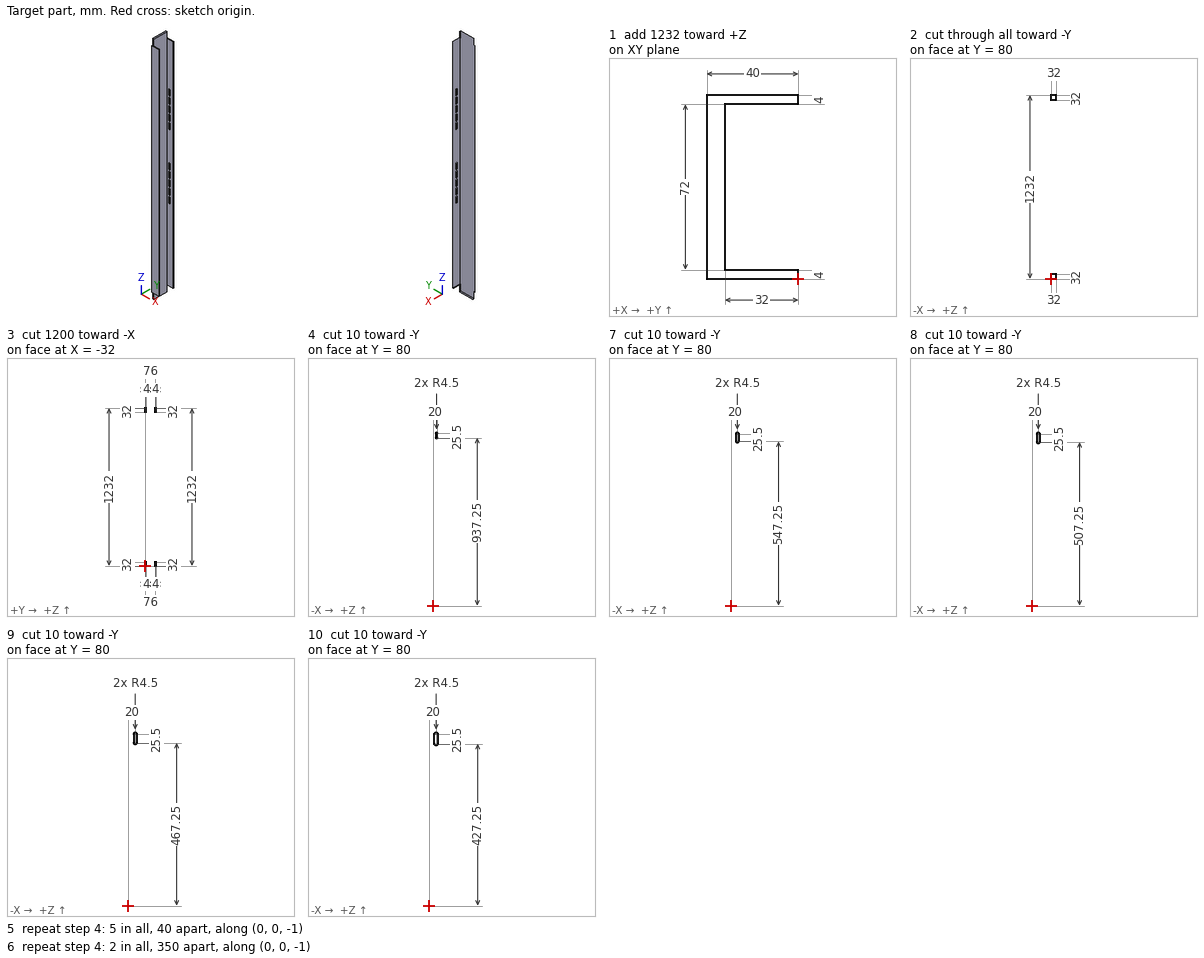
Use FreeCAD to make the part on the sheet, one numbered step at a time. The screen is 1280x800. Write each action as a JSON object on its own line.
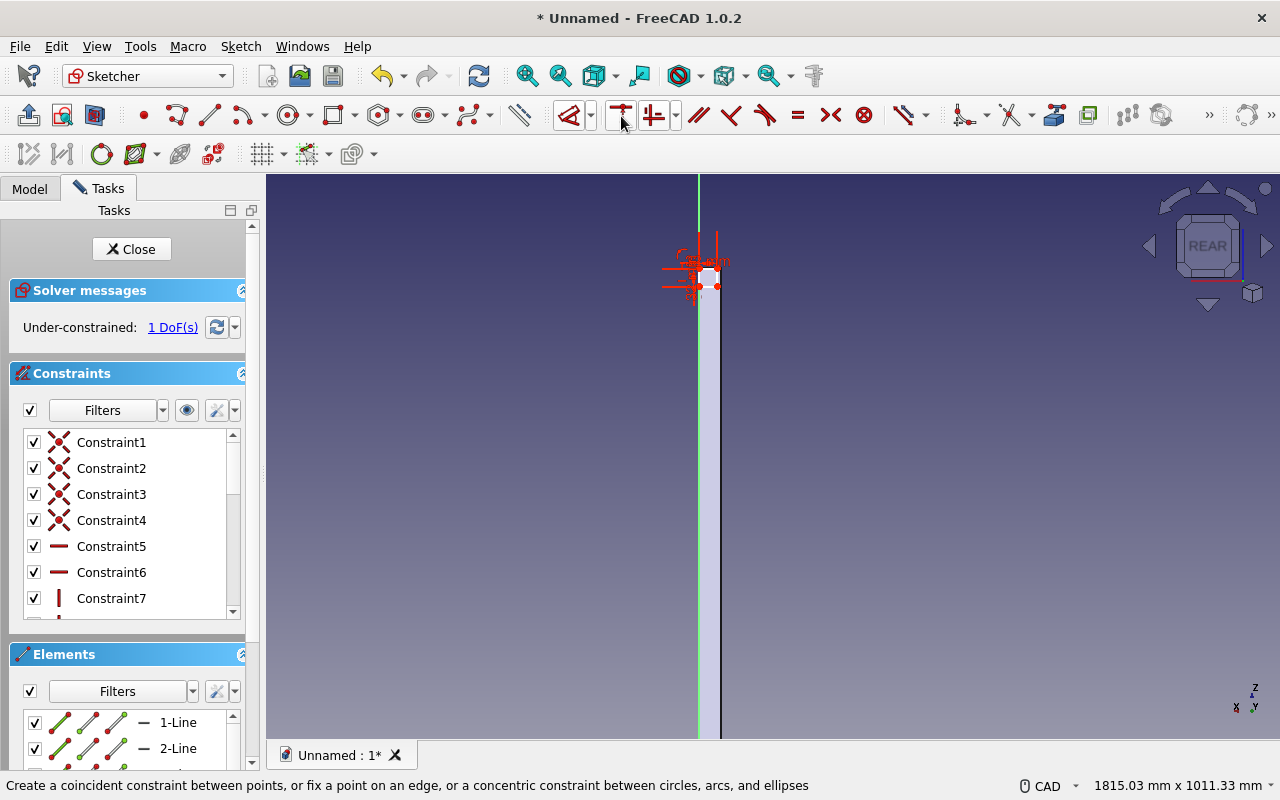
{"action": "left_click", "coordinate": [699, 269]}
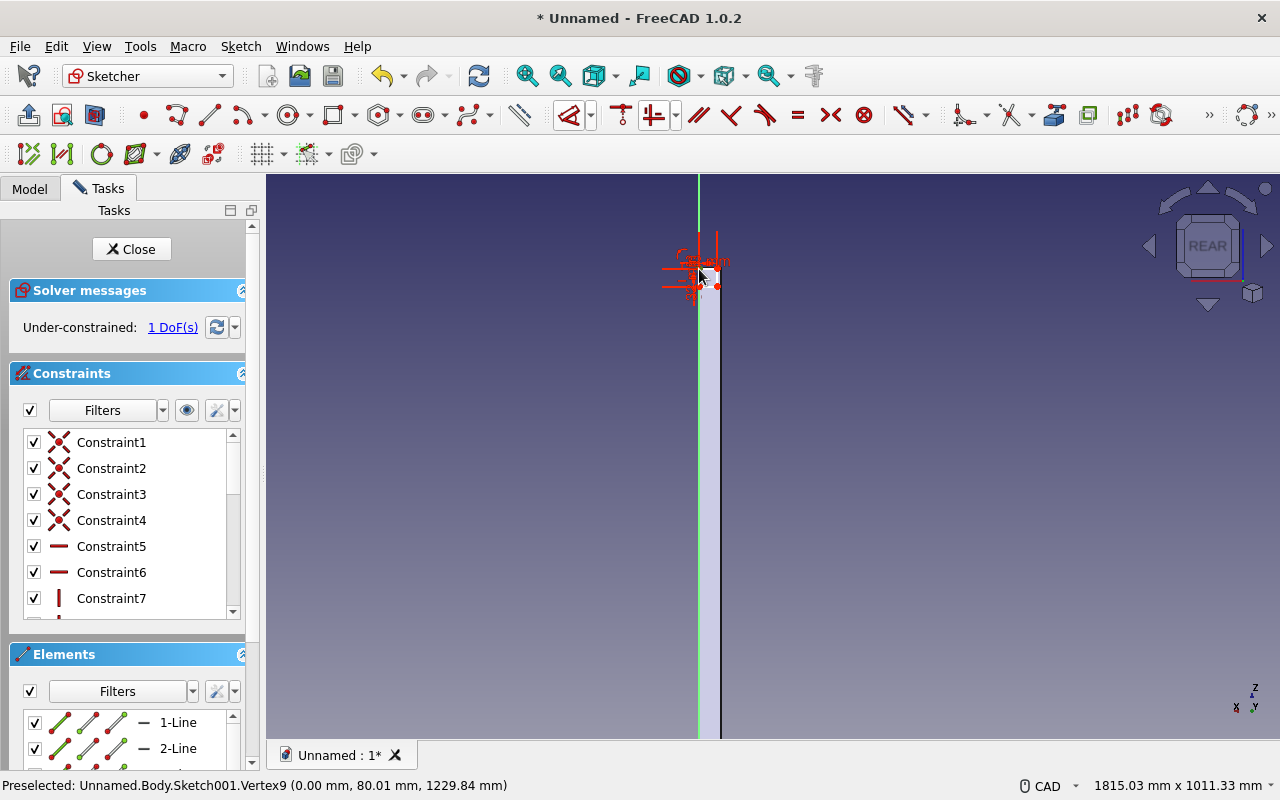
{"action": "left_click", "coordinate": [590, 116]}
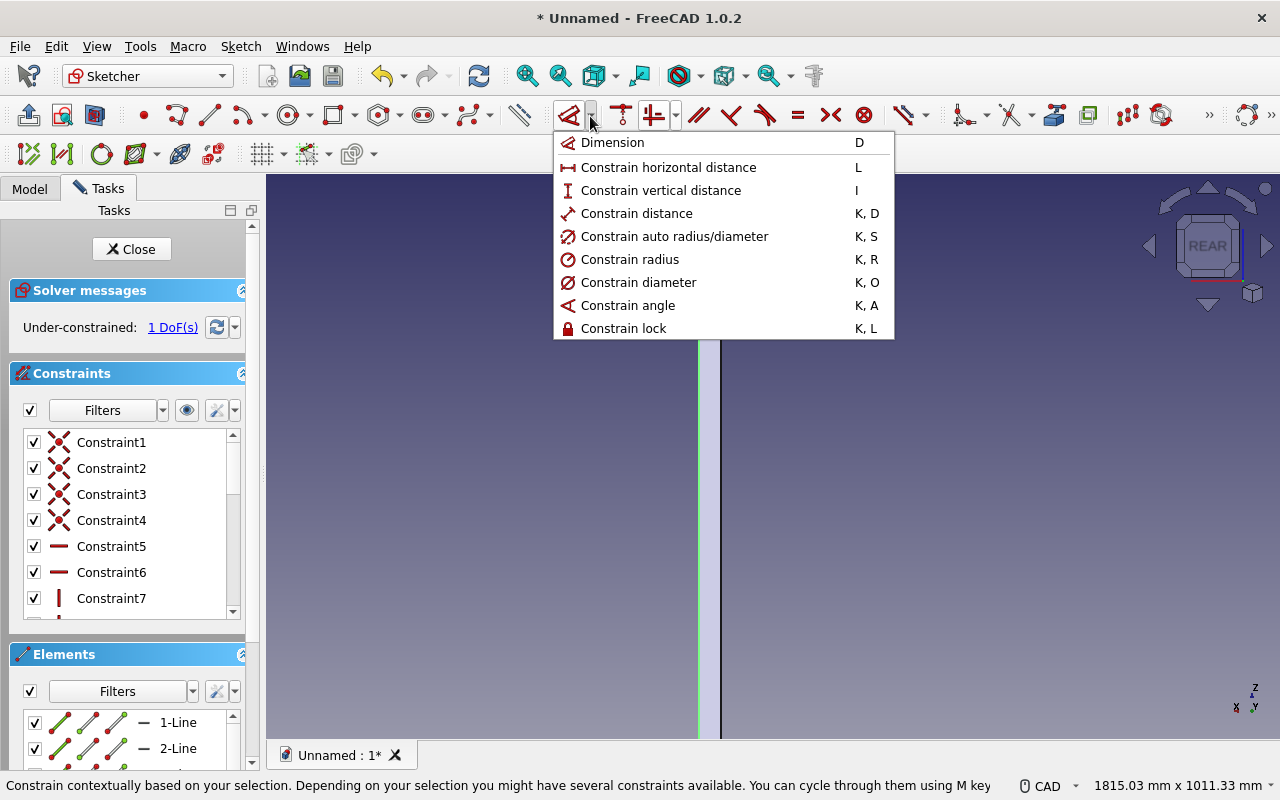
{"action": "left_click", "coordinate": [724, 190]}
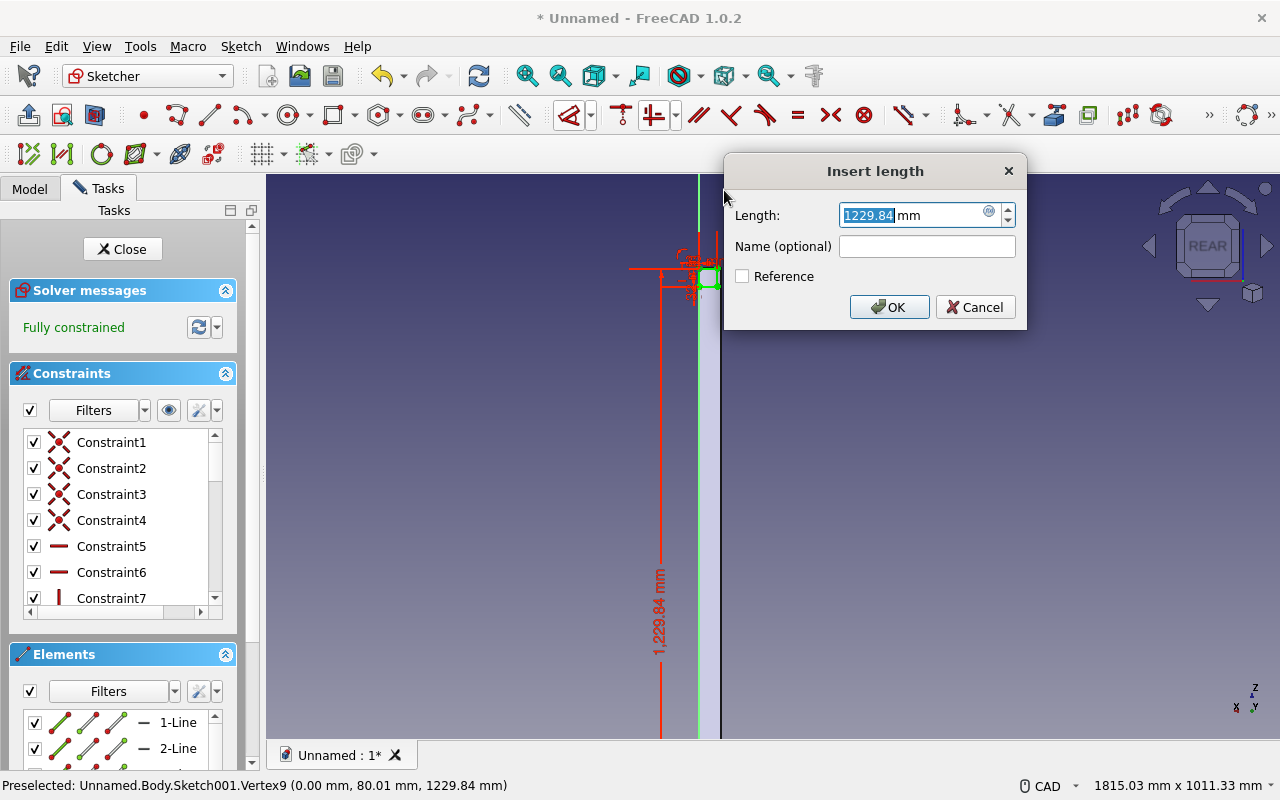
{"action": "type", "text": "1232"}
{"action": "key", "text": "Return"}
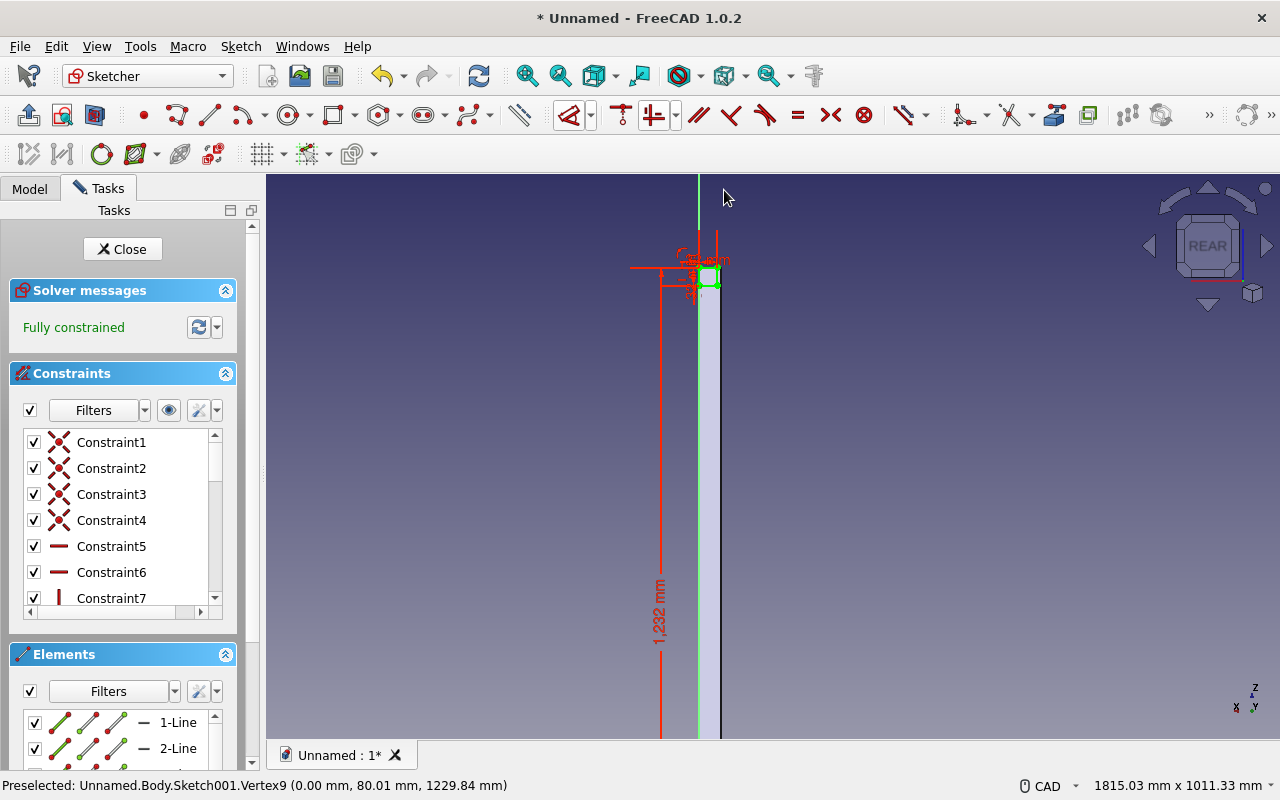
{"action": "left_click", "coordinate": [123, 249]}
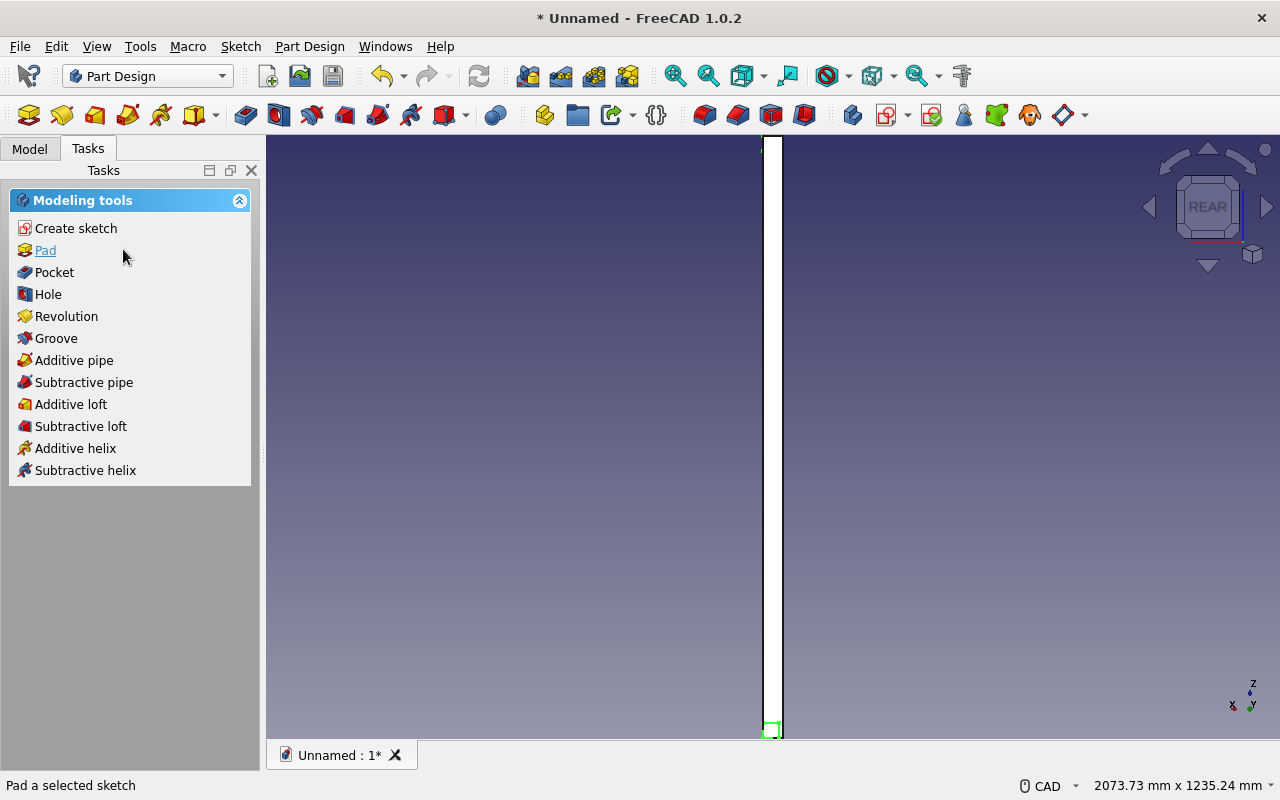
{"action": "left_click", "coordinate": [246, 116]}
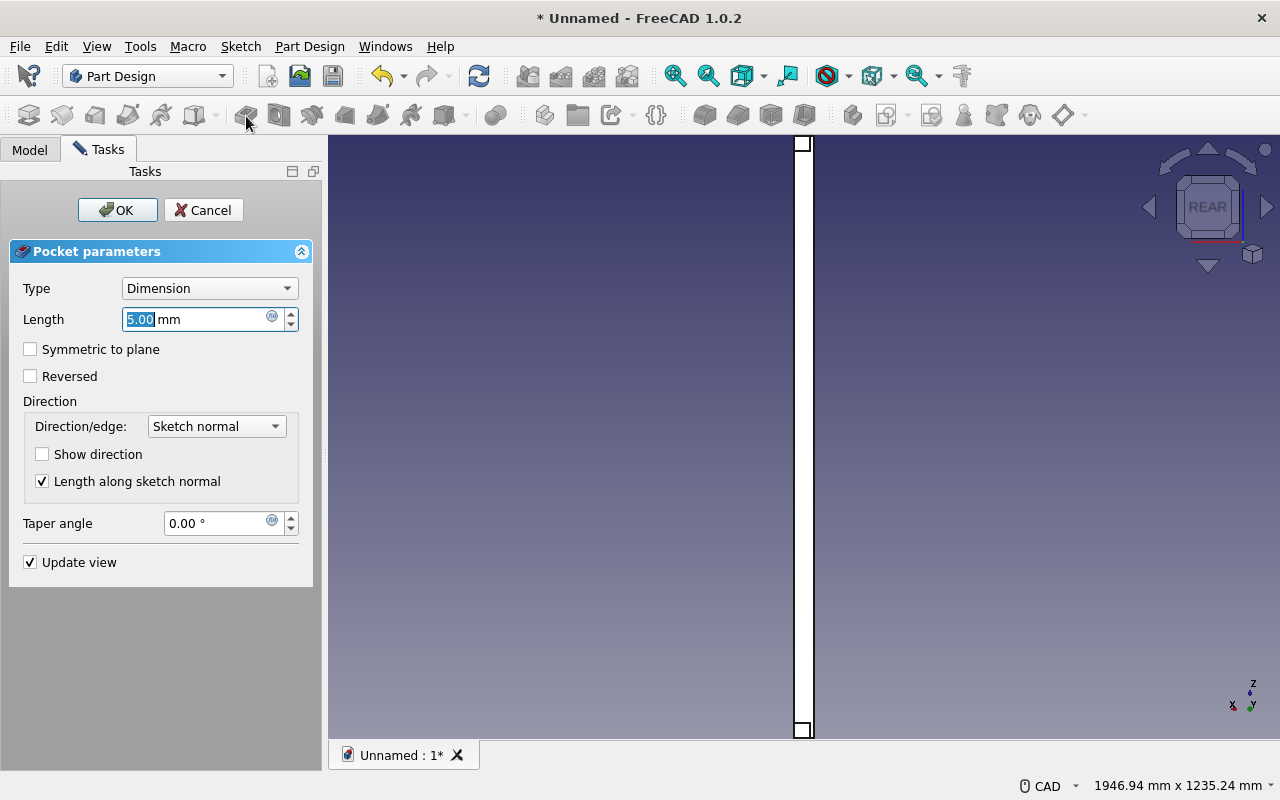
{"action": "left_click", "coordinate": [210, 288]}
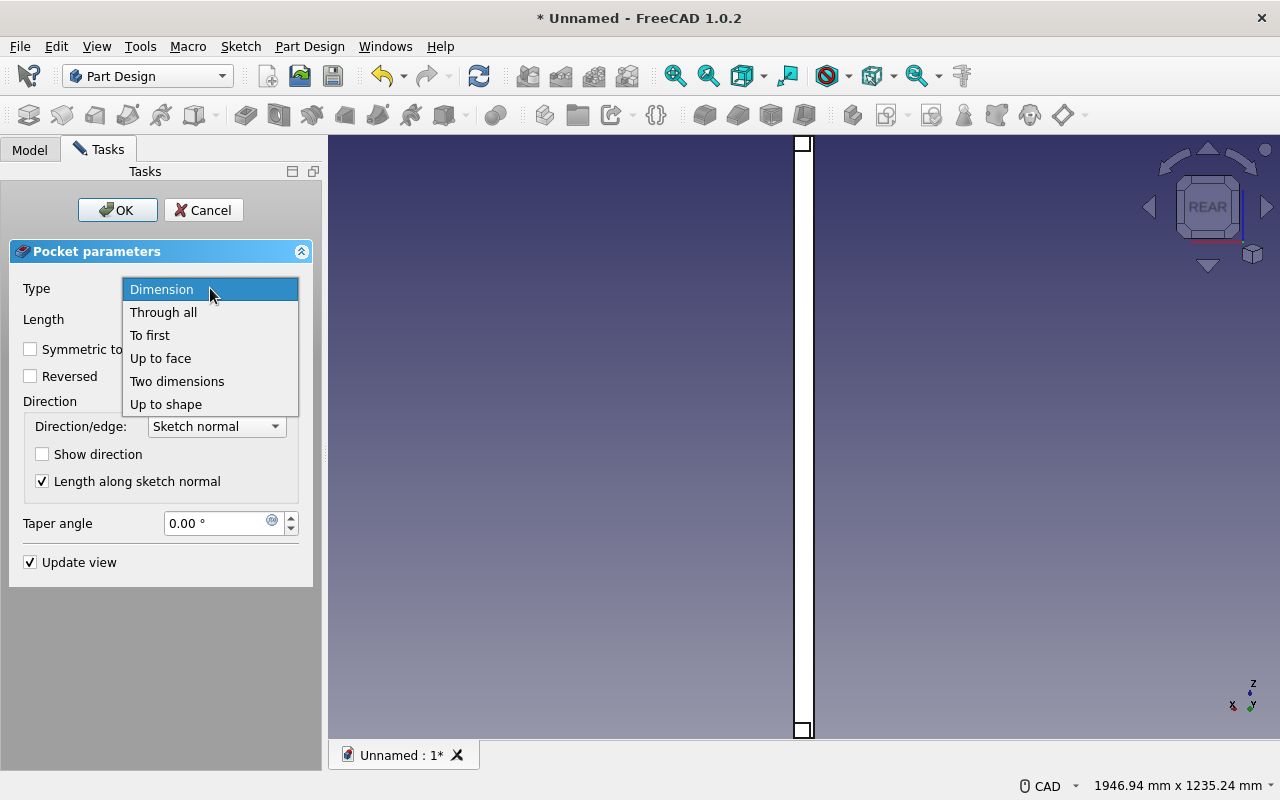
{"action": "left_click", "coordinate": [208, 312]}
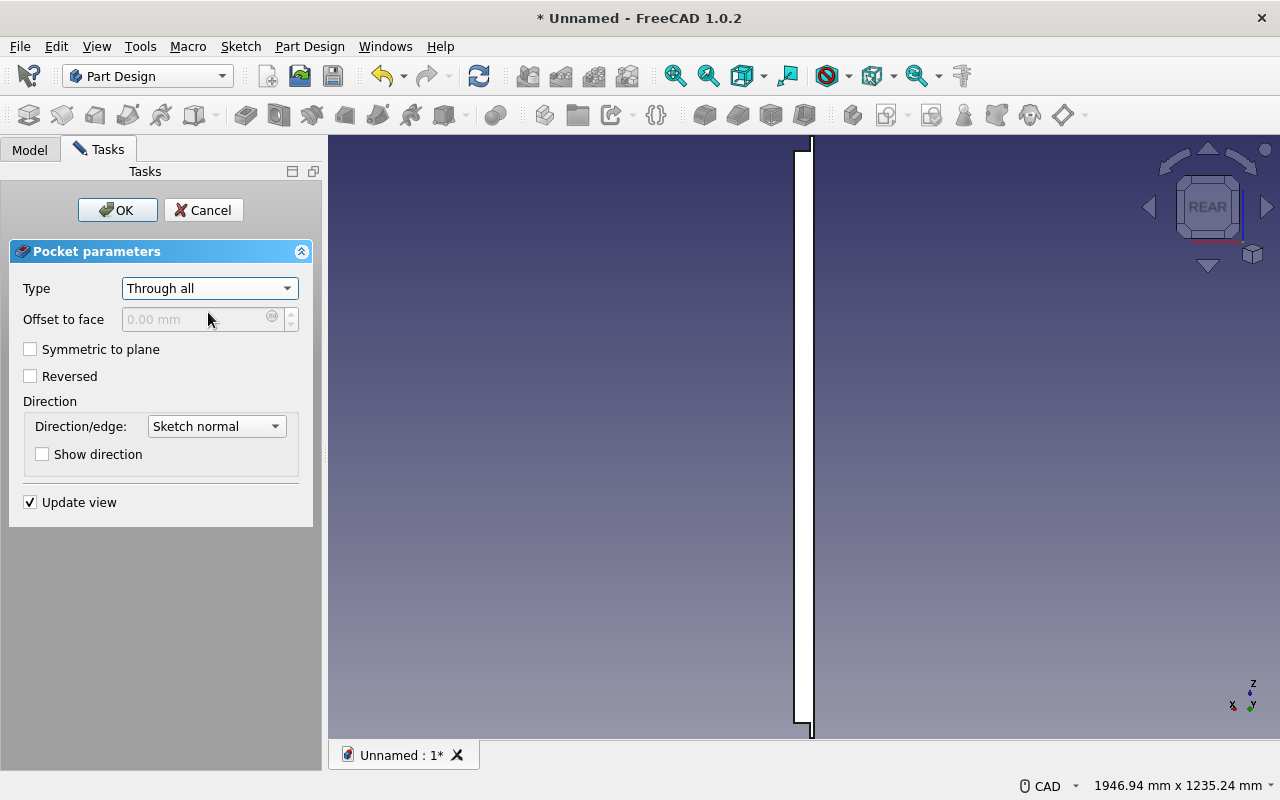
{"action": "left_click", "coordinate": [118, 210]}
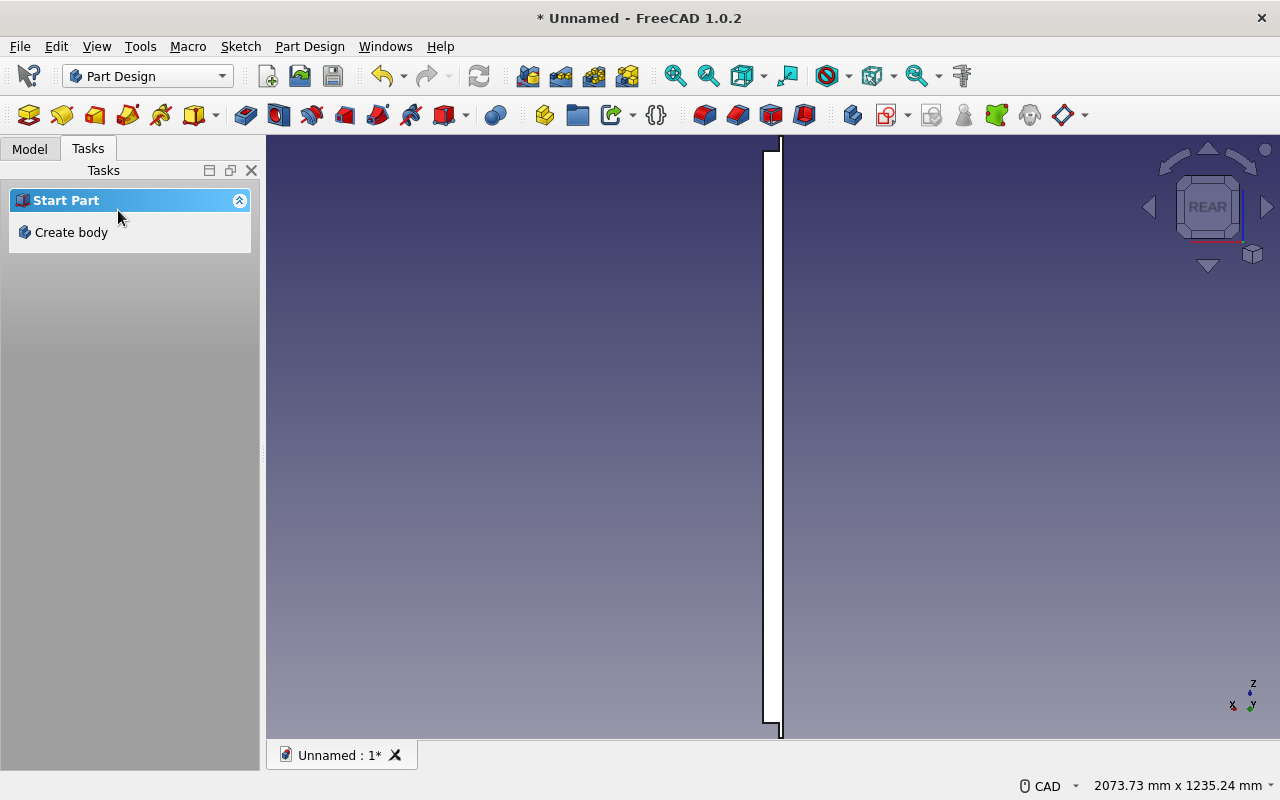
{"action": "key", "text": "0"}